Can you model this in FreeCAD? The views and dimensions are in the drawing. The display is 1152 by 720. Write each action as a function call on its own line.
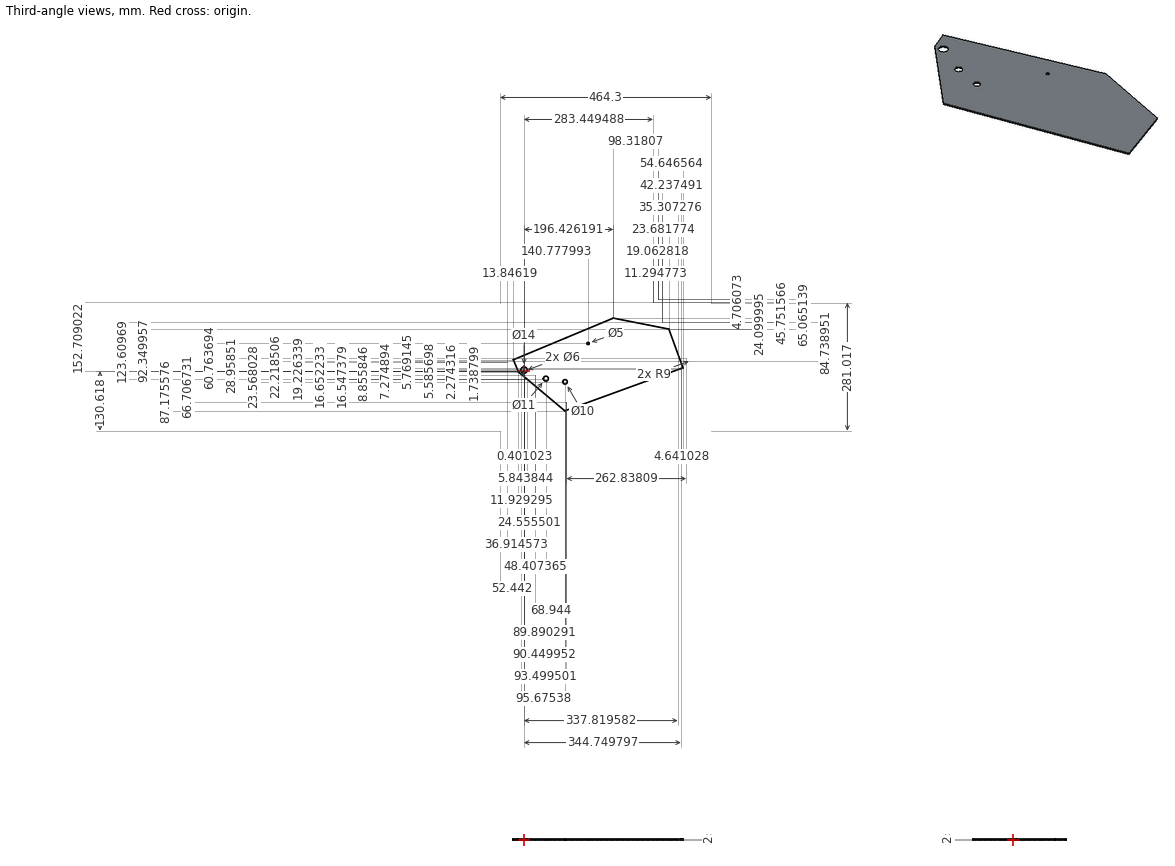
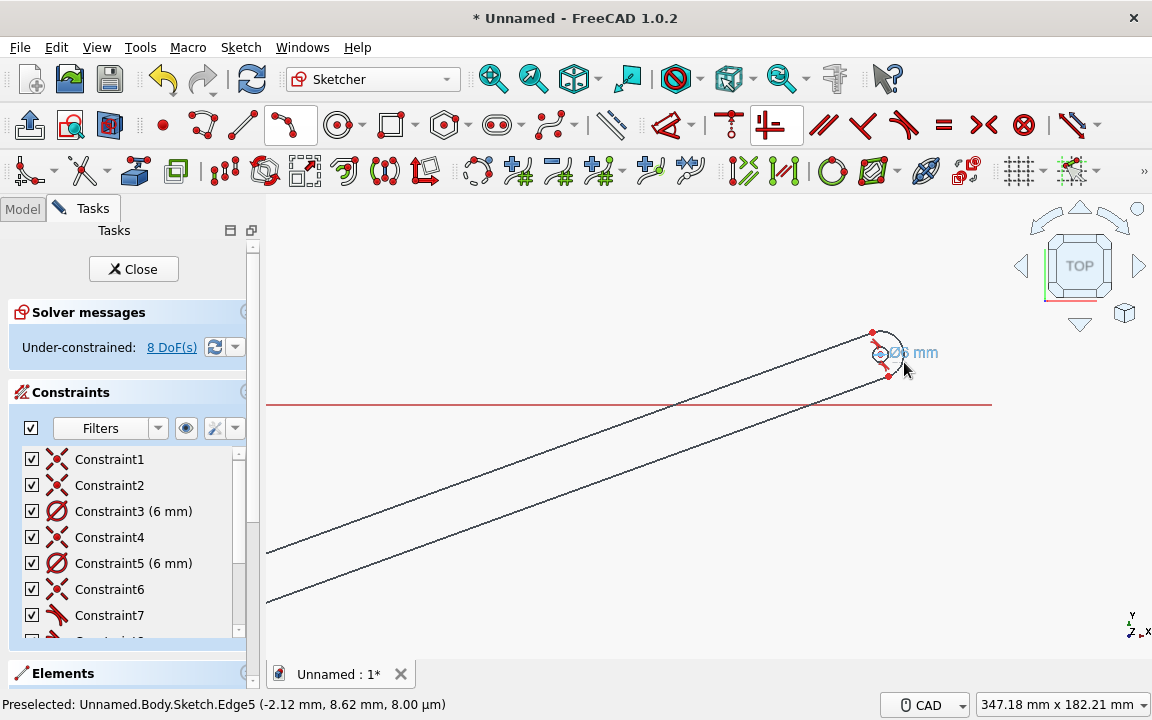
click(903, 361)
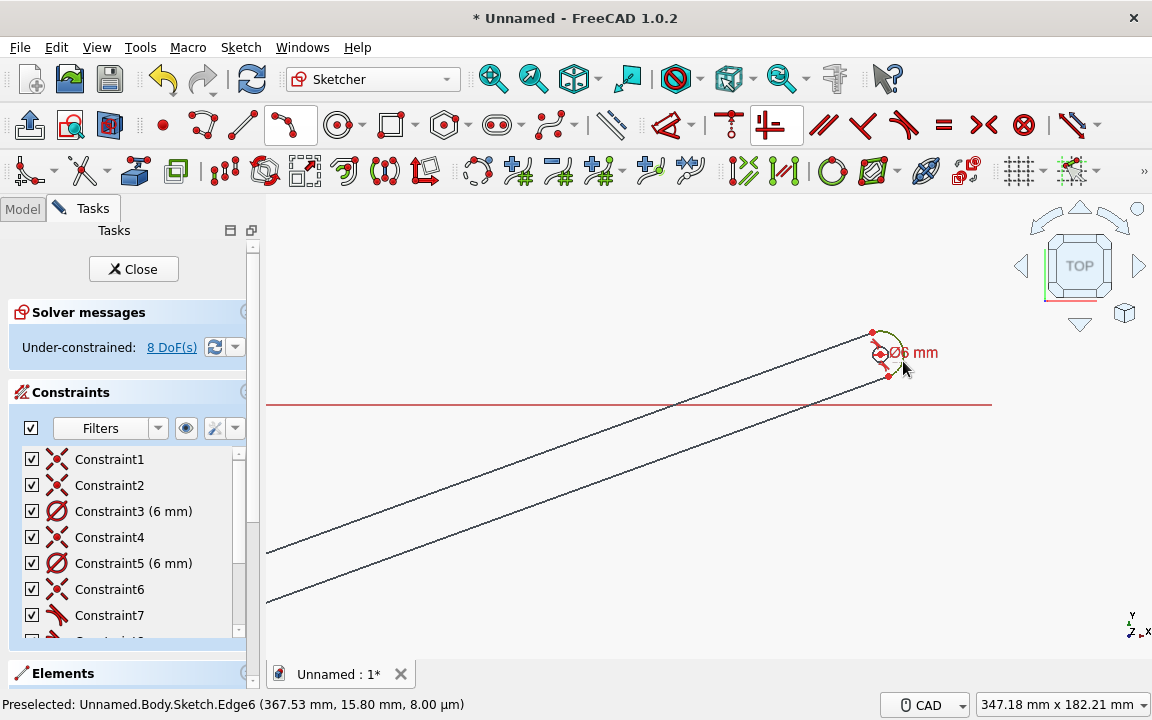
key(e)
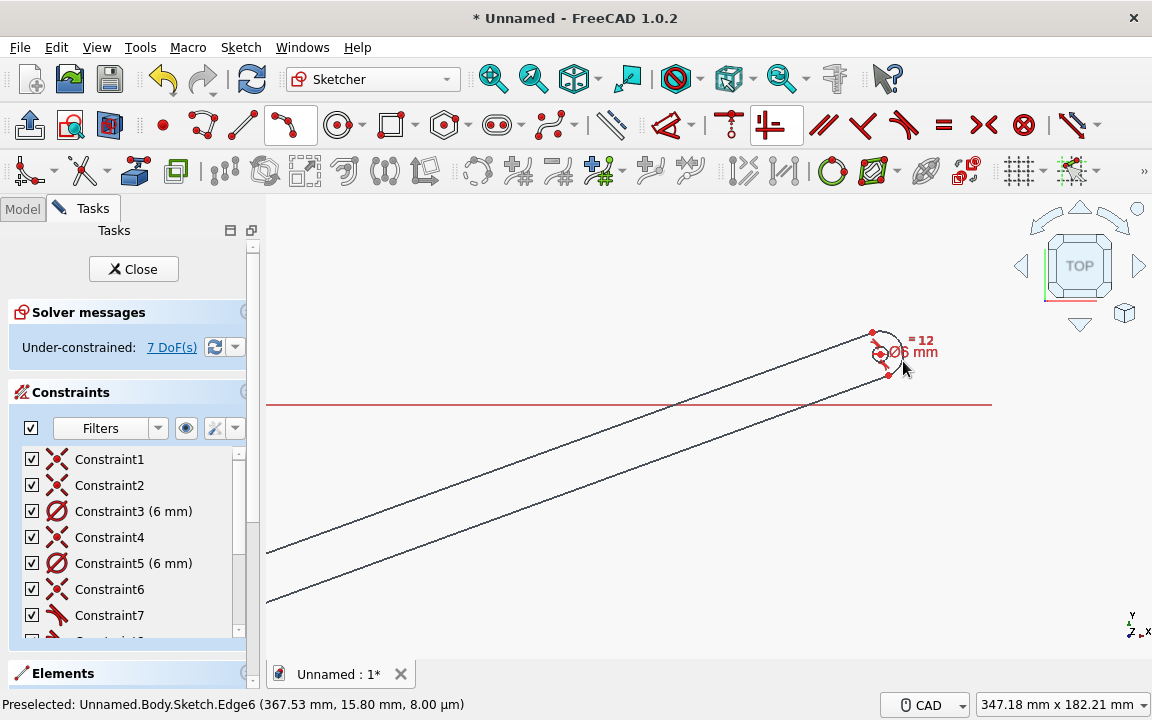
scroll(904, 362, down, 3)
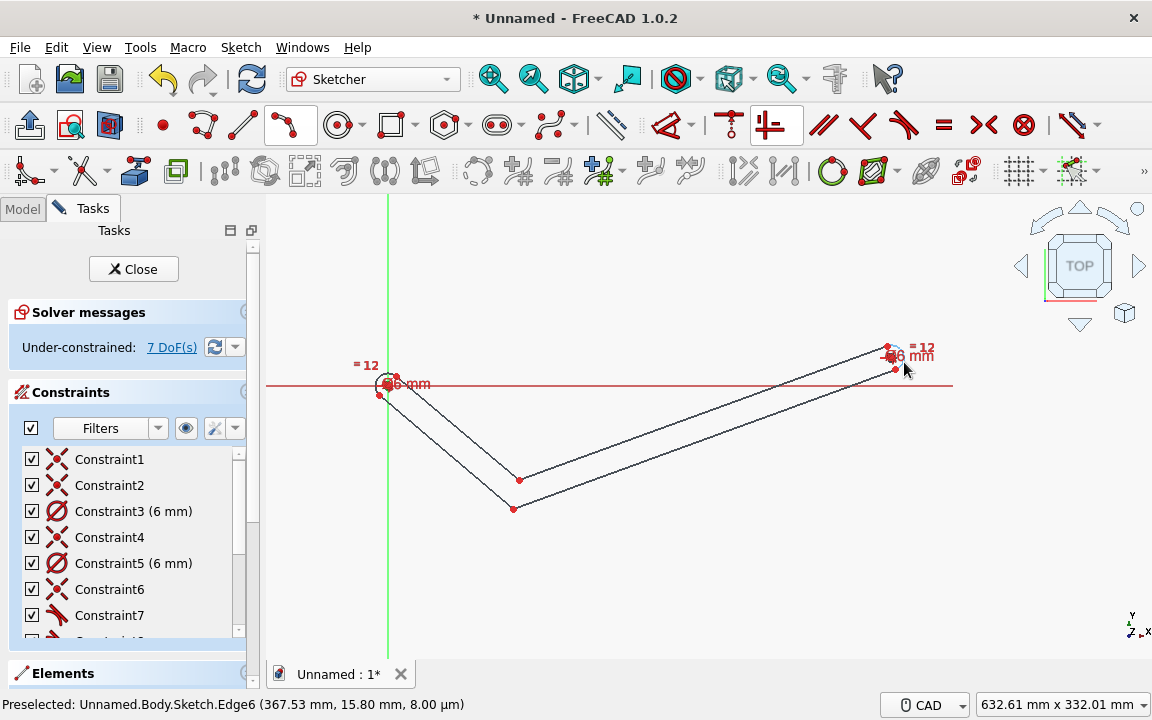
scroll(376, 385, up, 6)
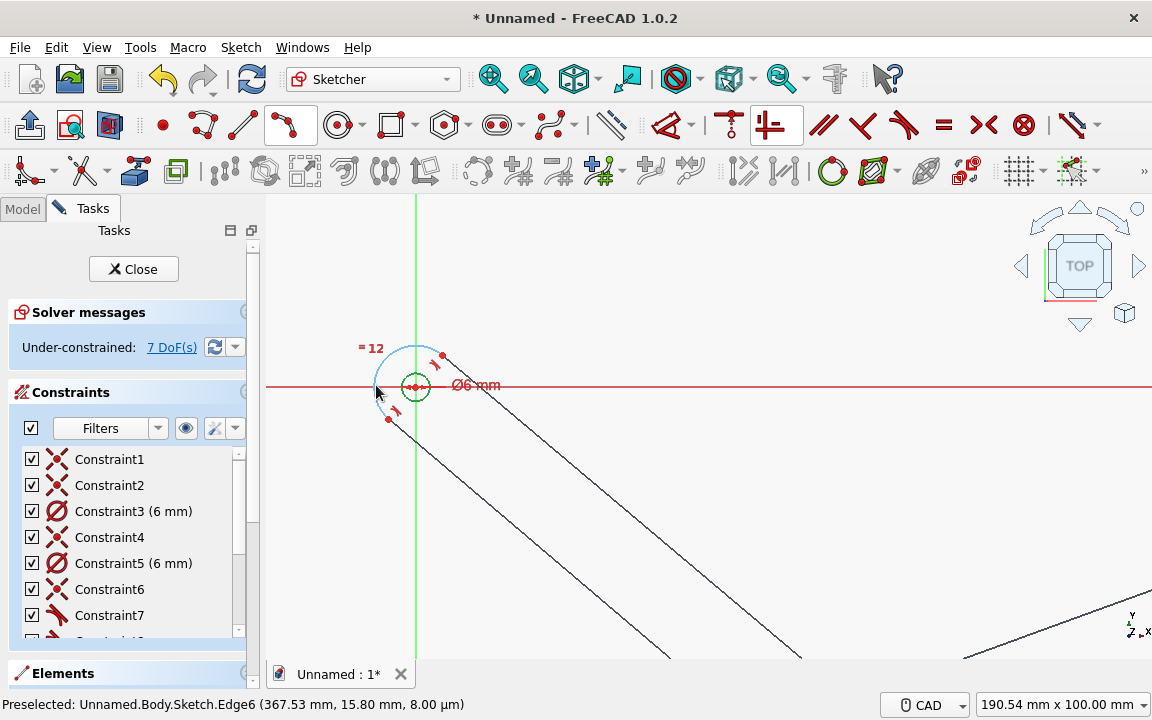
click(374, 384)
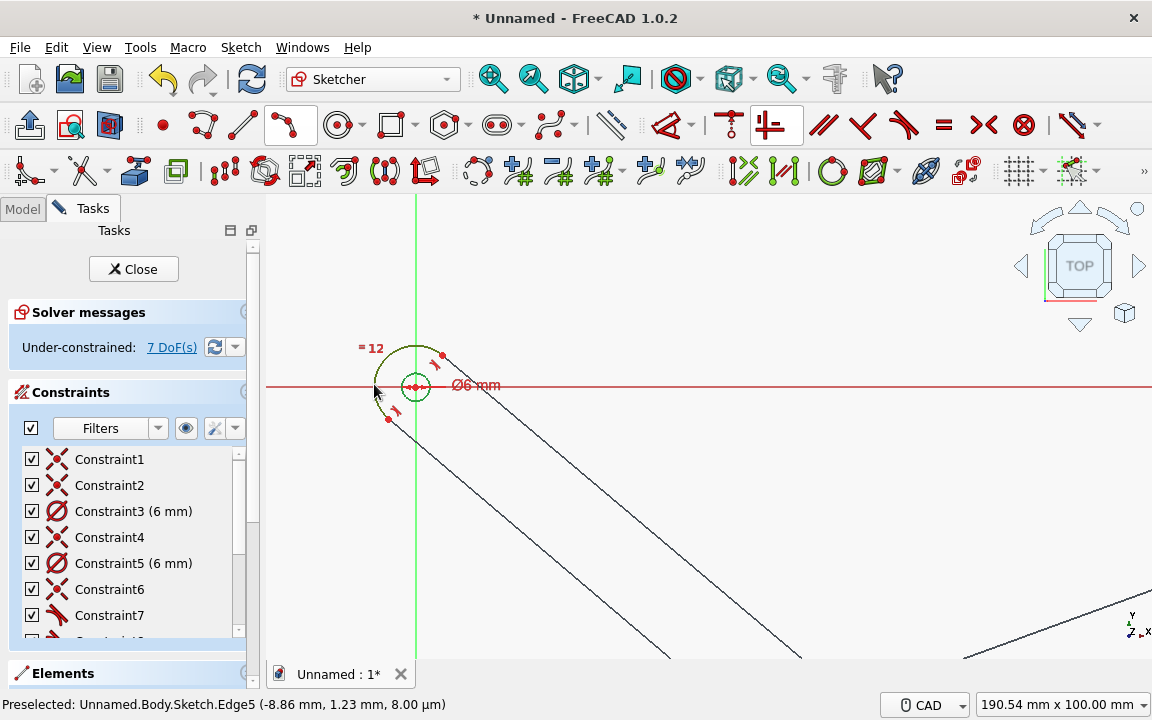
key(k)
key(r)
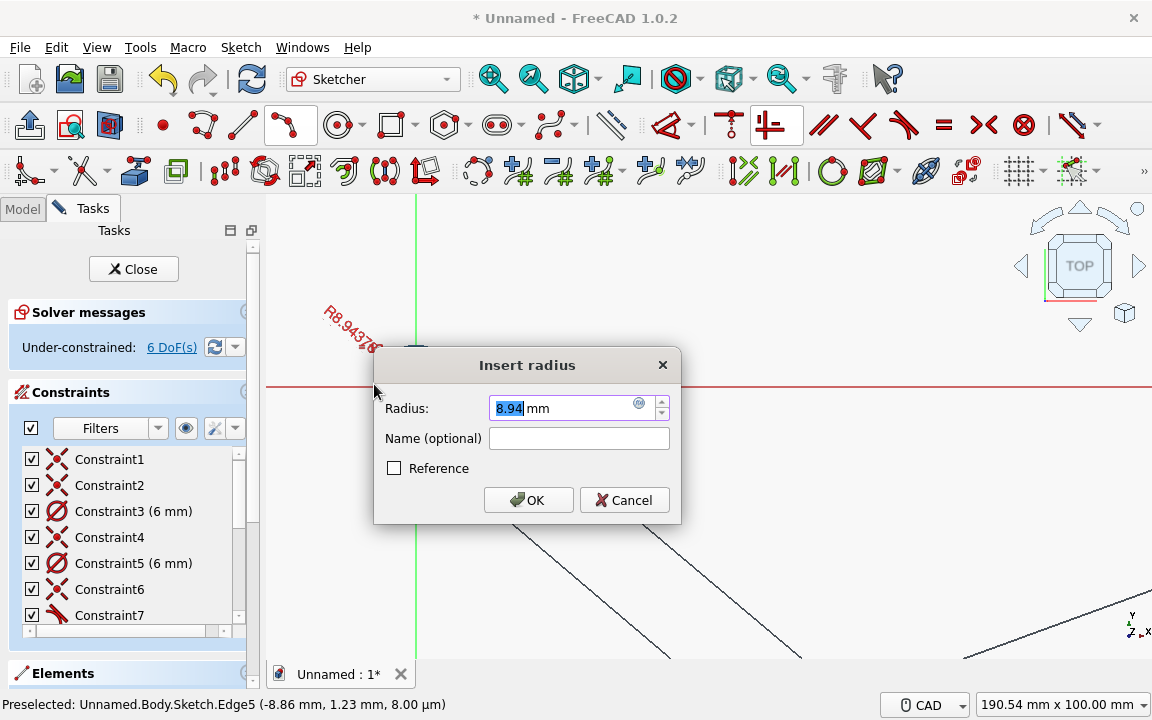
text(9)
key(Return)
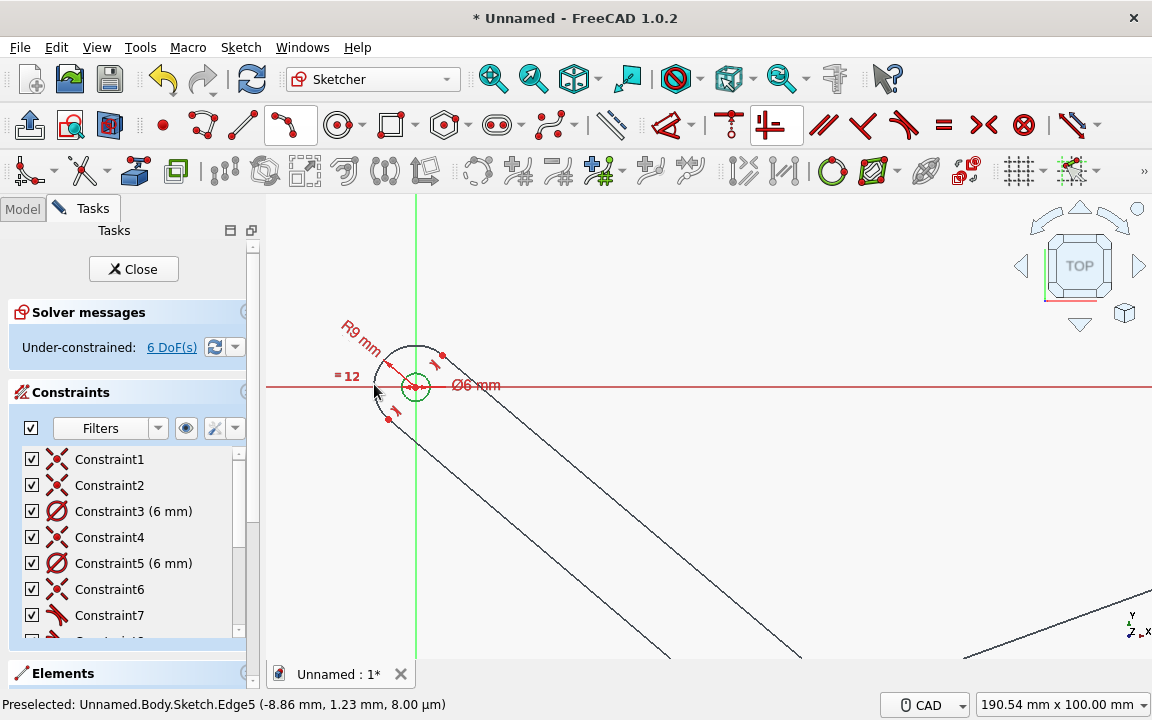
scroll(376, 385, down, 6)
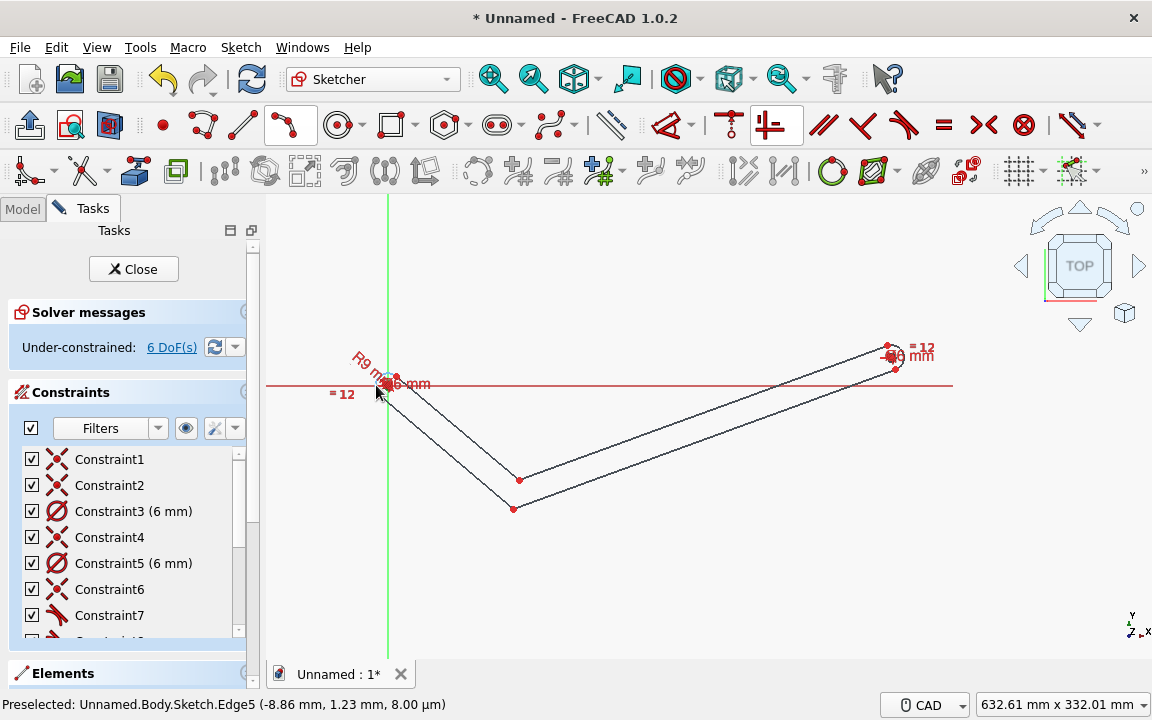
click(887, 346)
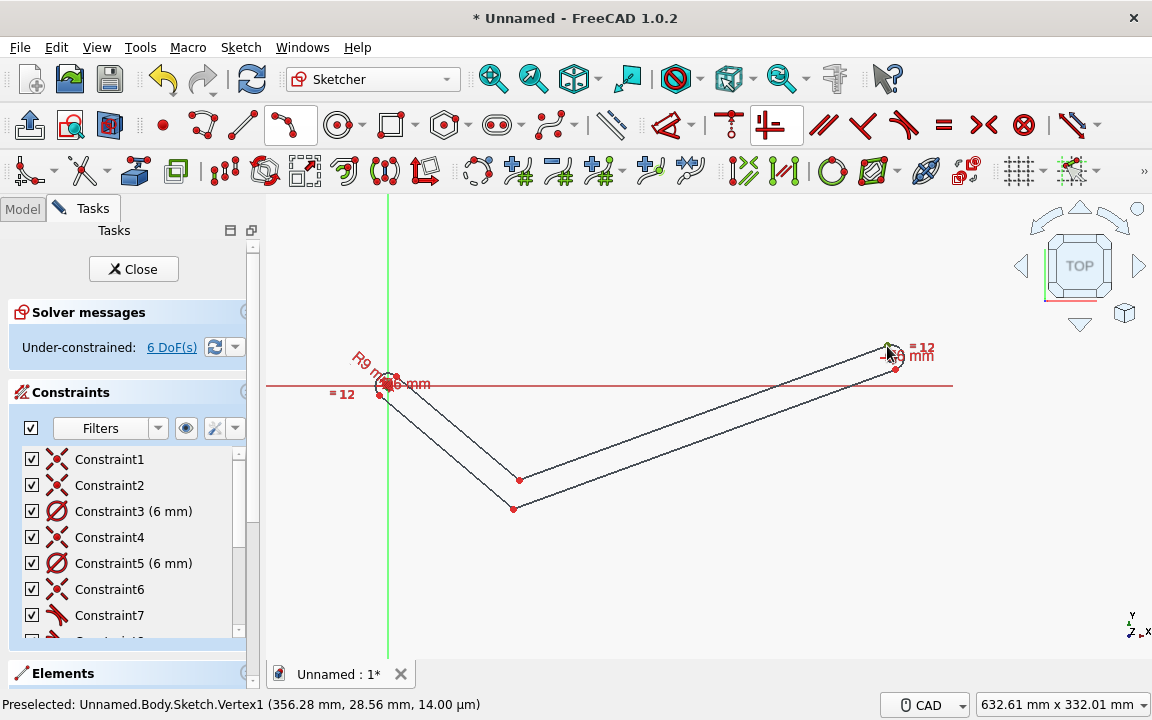
key(i)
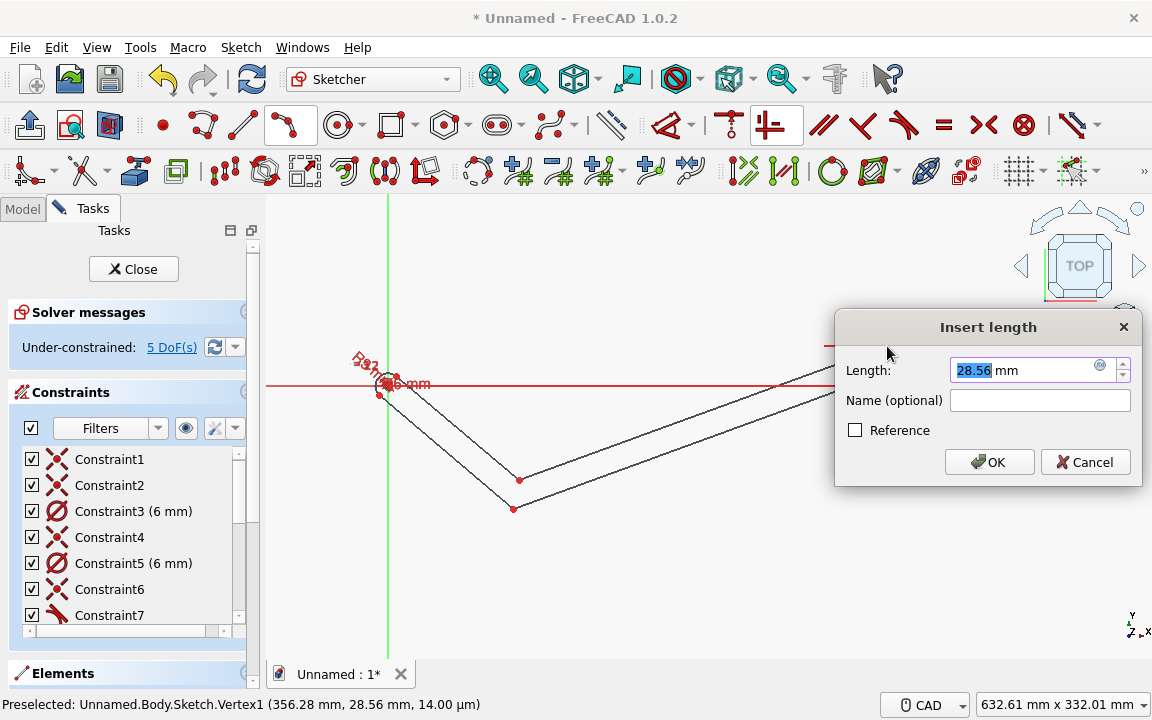
text(28.95851)
key(Return)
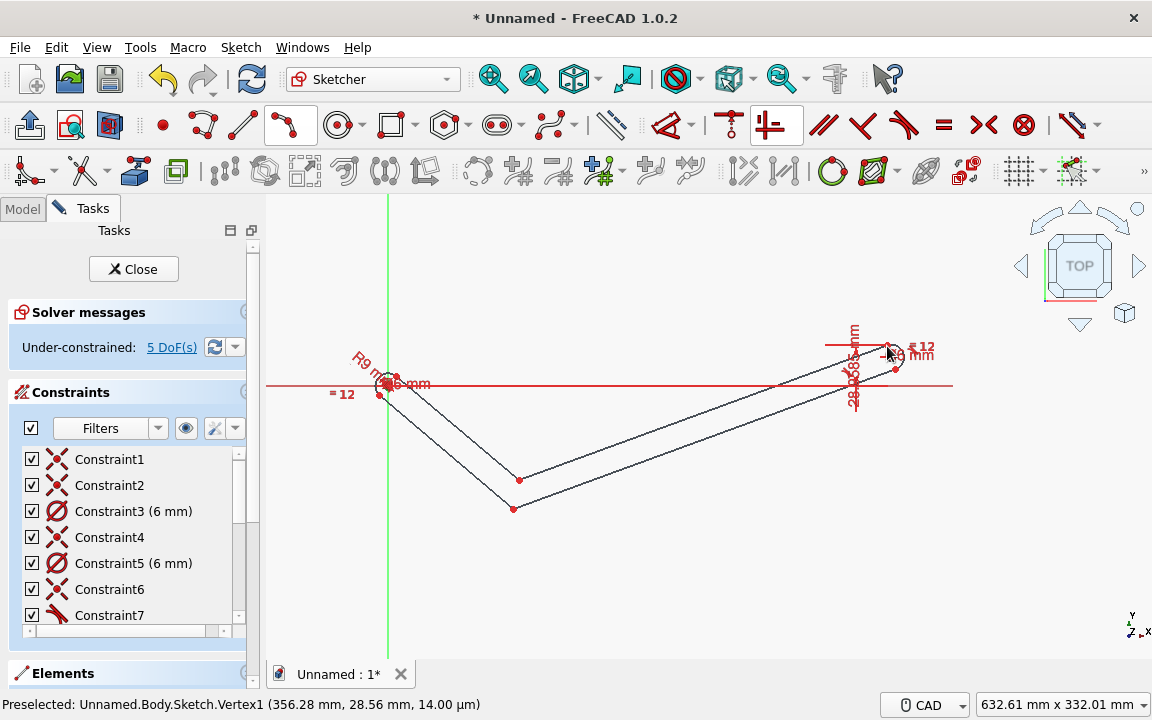
click(420, 430)